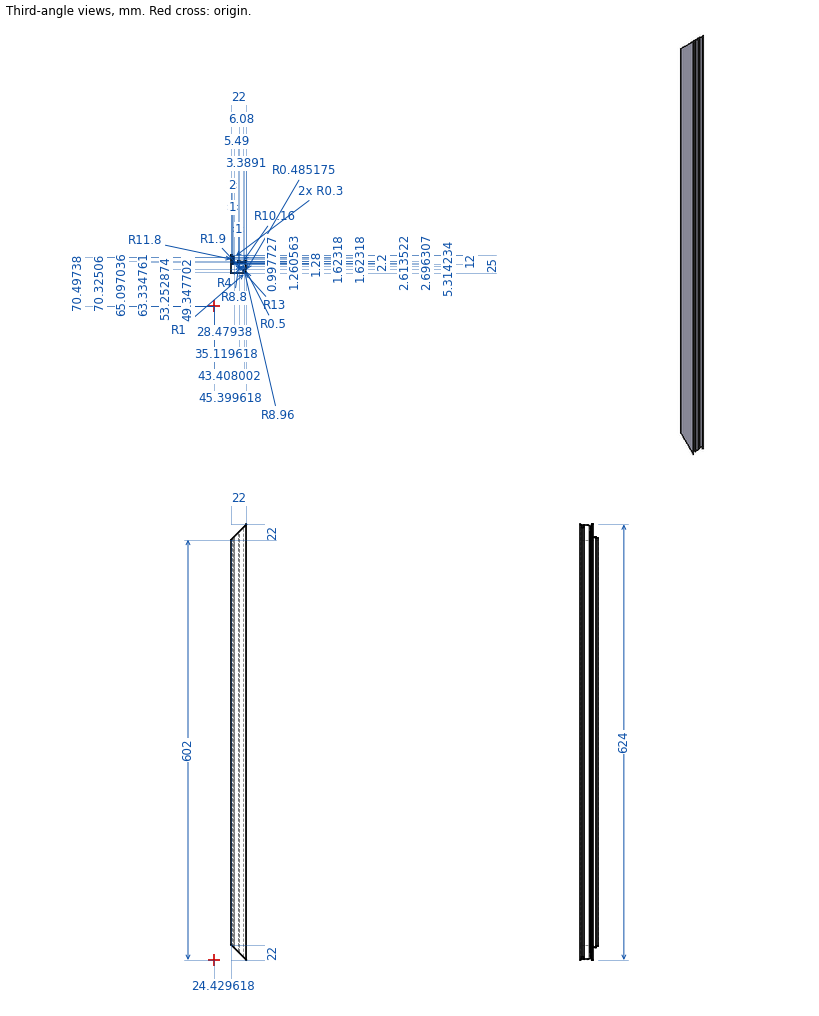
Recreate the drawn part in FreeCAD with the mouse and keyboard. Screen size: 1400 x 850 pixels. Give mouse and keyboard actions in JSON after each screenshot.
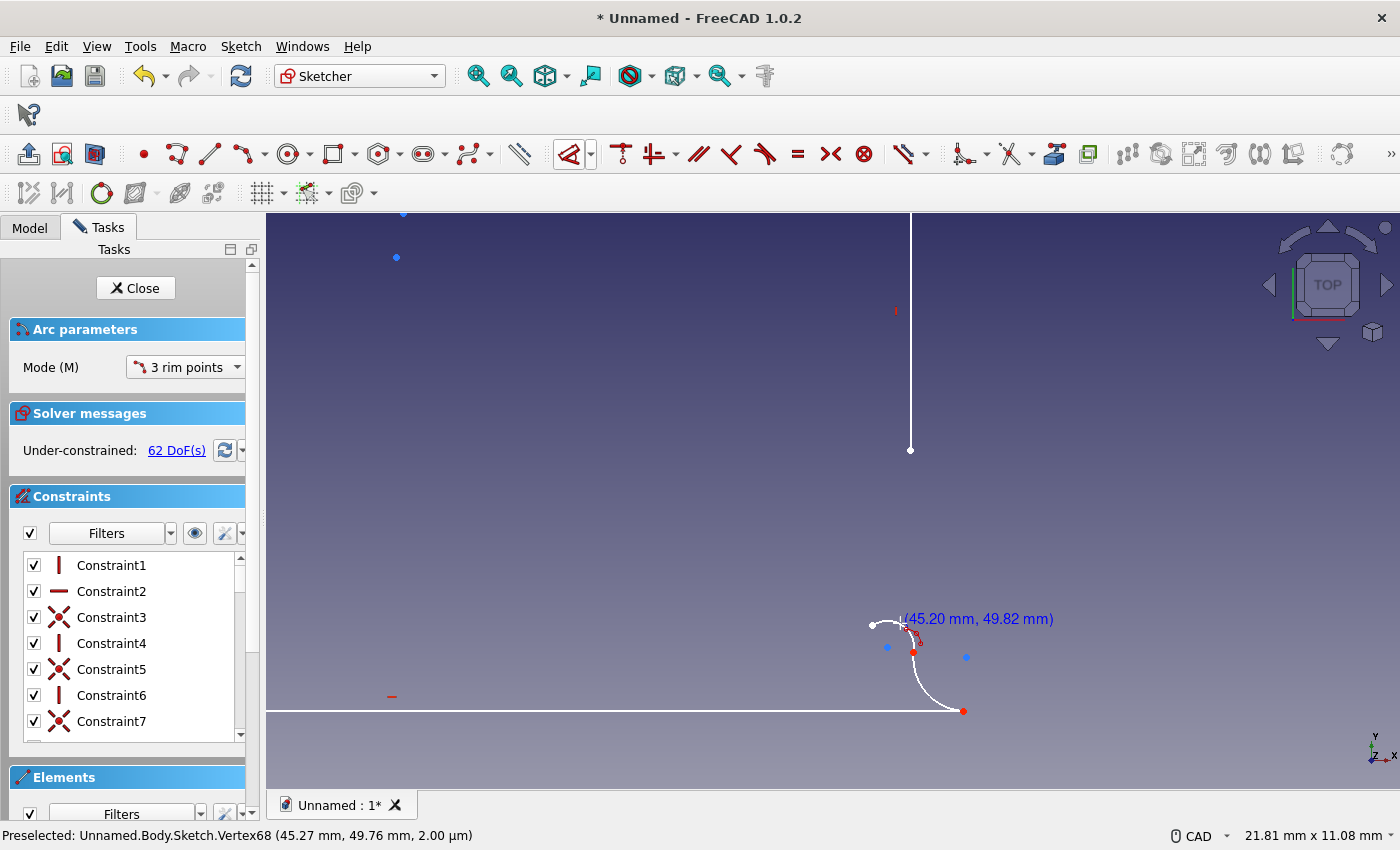
{"action": "left_click", "coordinate": [872, 626]}
{"action": "left_click", "coordinate": [869, 467]}
{"action": "left_click", "coordinate": [713, 549]}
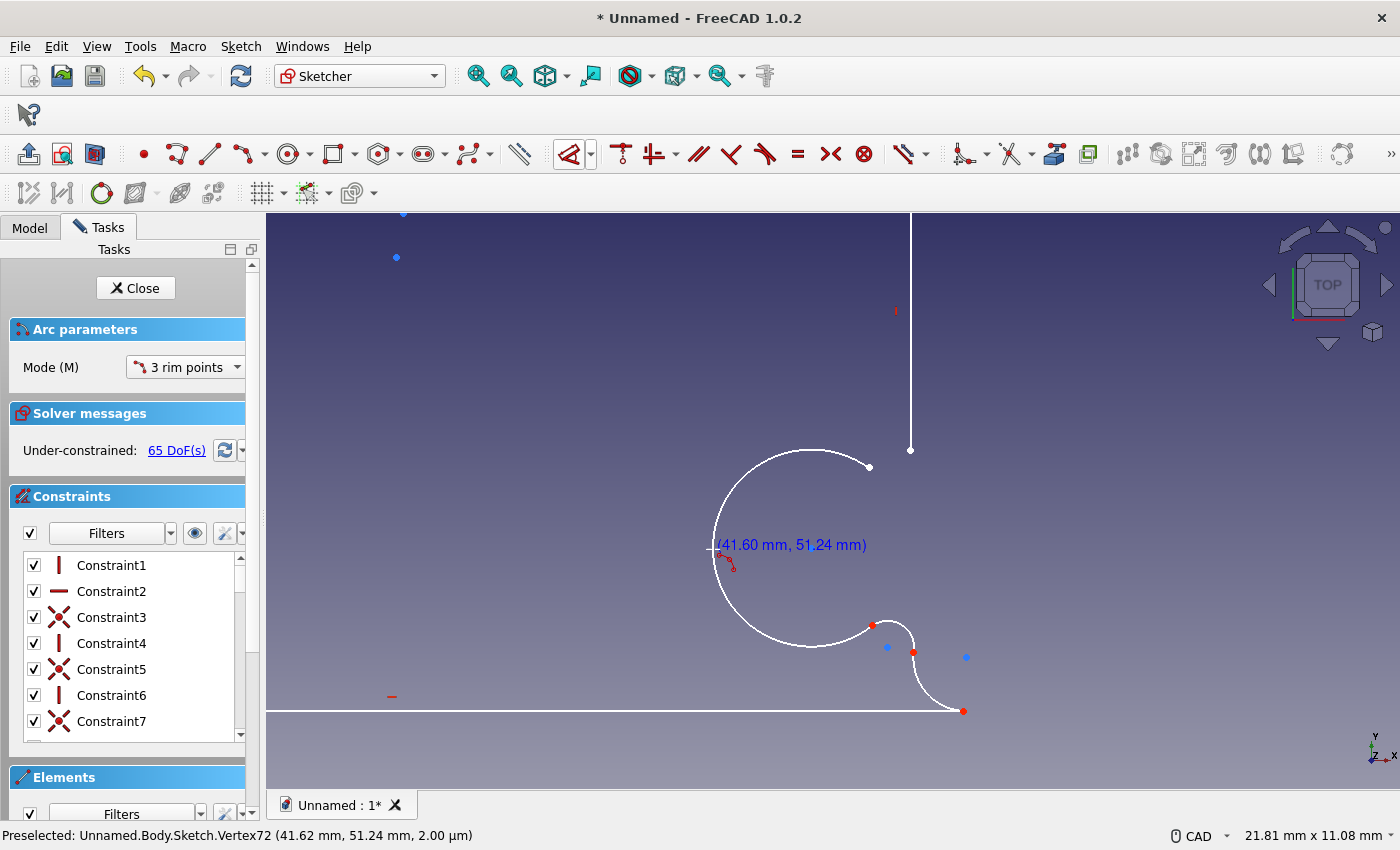
{"action": "left_click", "coordinate": [869, 468]}
{"action": "left_click", "coordinate": [911, 450]}
{"action": "left_click", "coordinate": [896, 469]}
{"action": "key", "text": "Escape"}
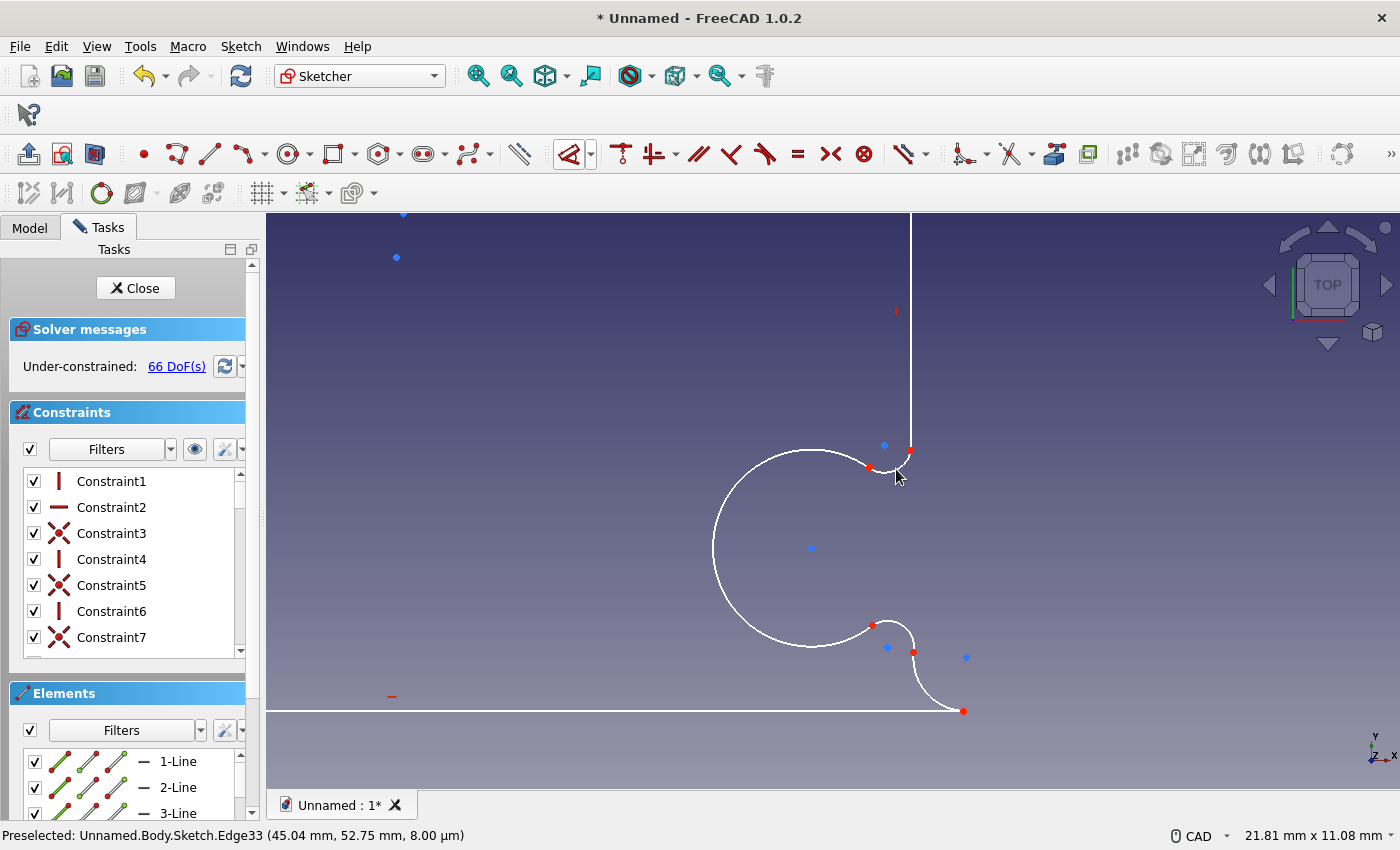
{"action": "left_click", "coordinate": [911, 366]}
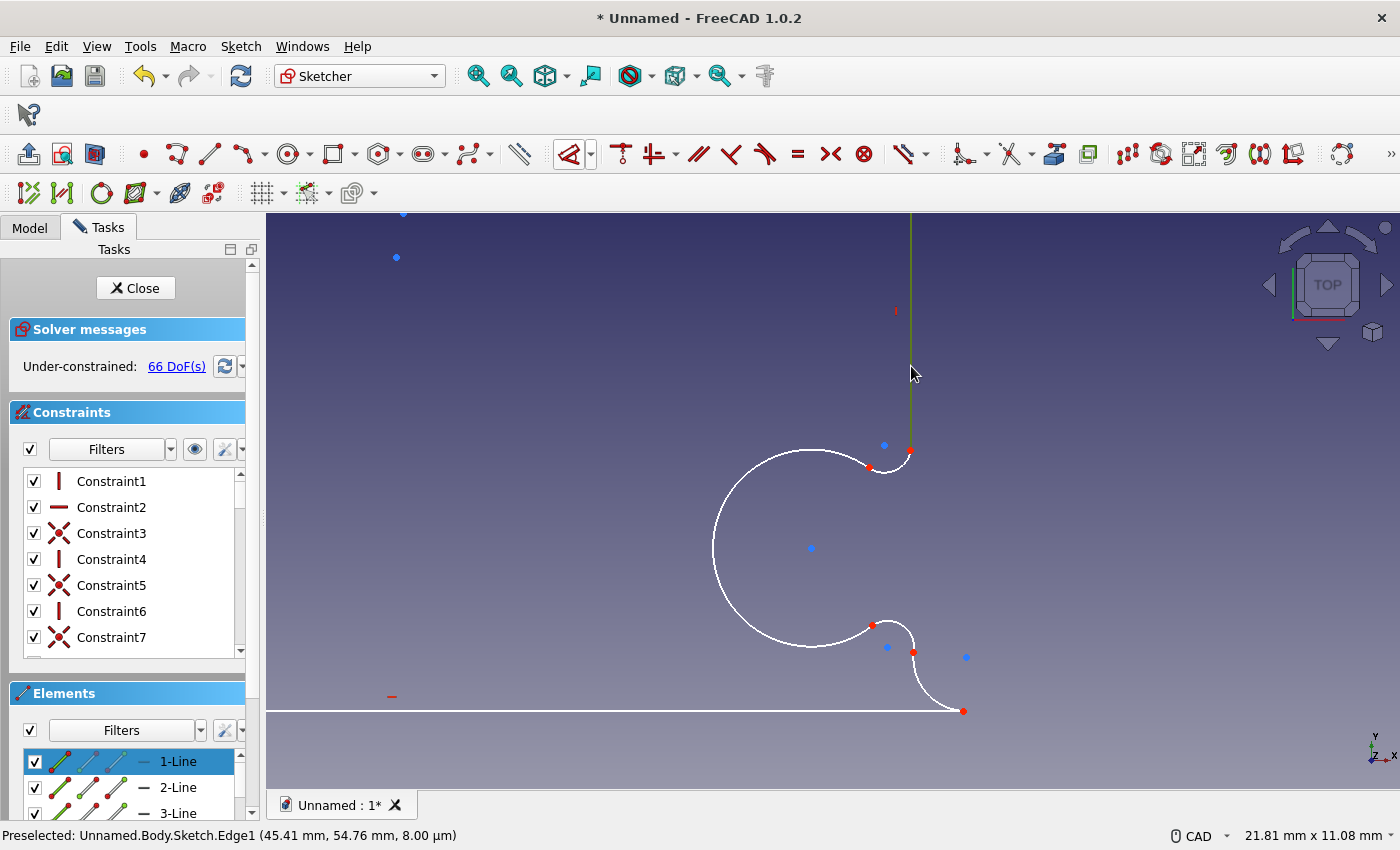
{"action": "scroll", "coordinate": [925, 692], "scroll_direction": "down", "scroll_amount": 6}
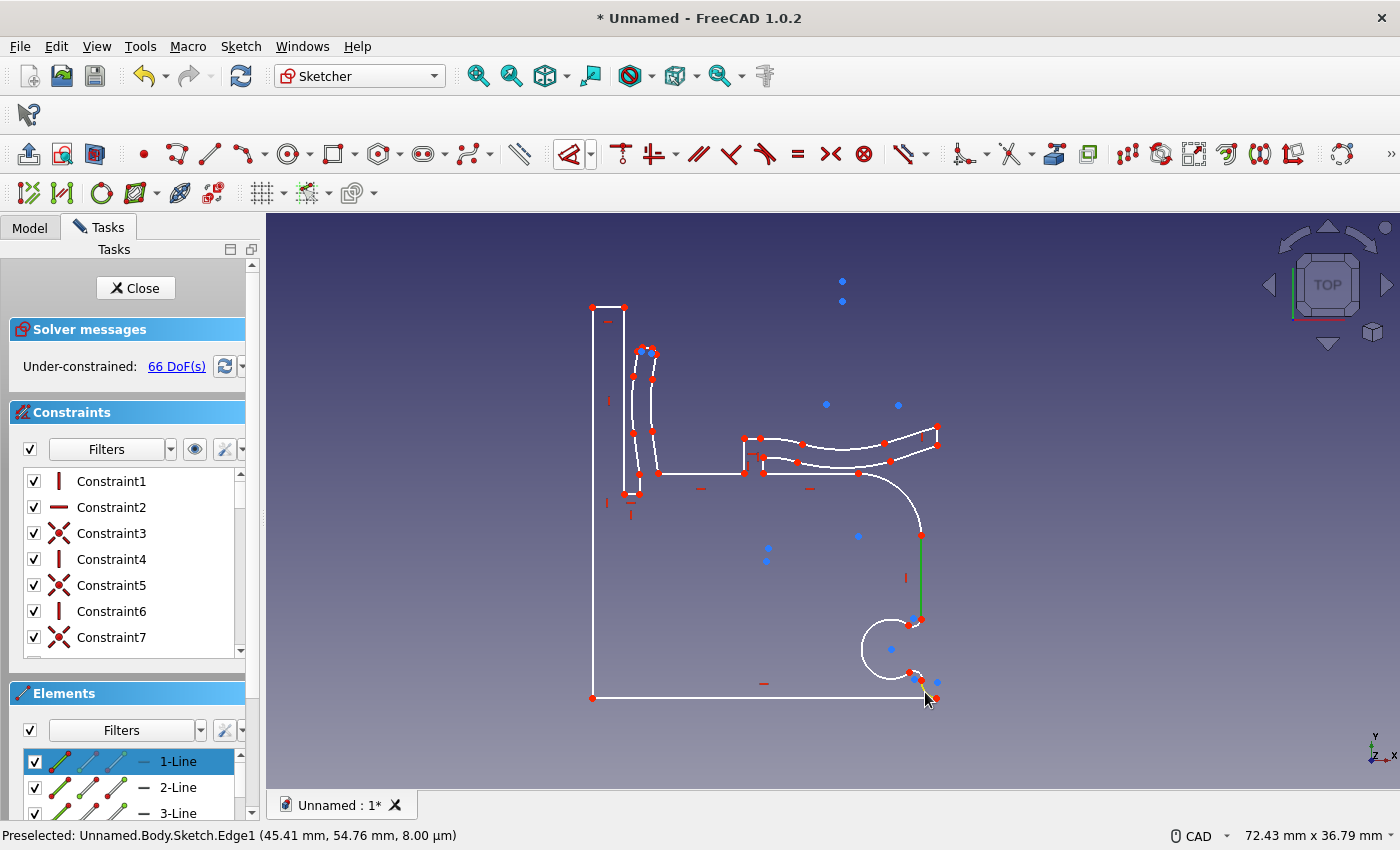
{"action": "left_click", "coordinate": [914, 507]}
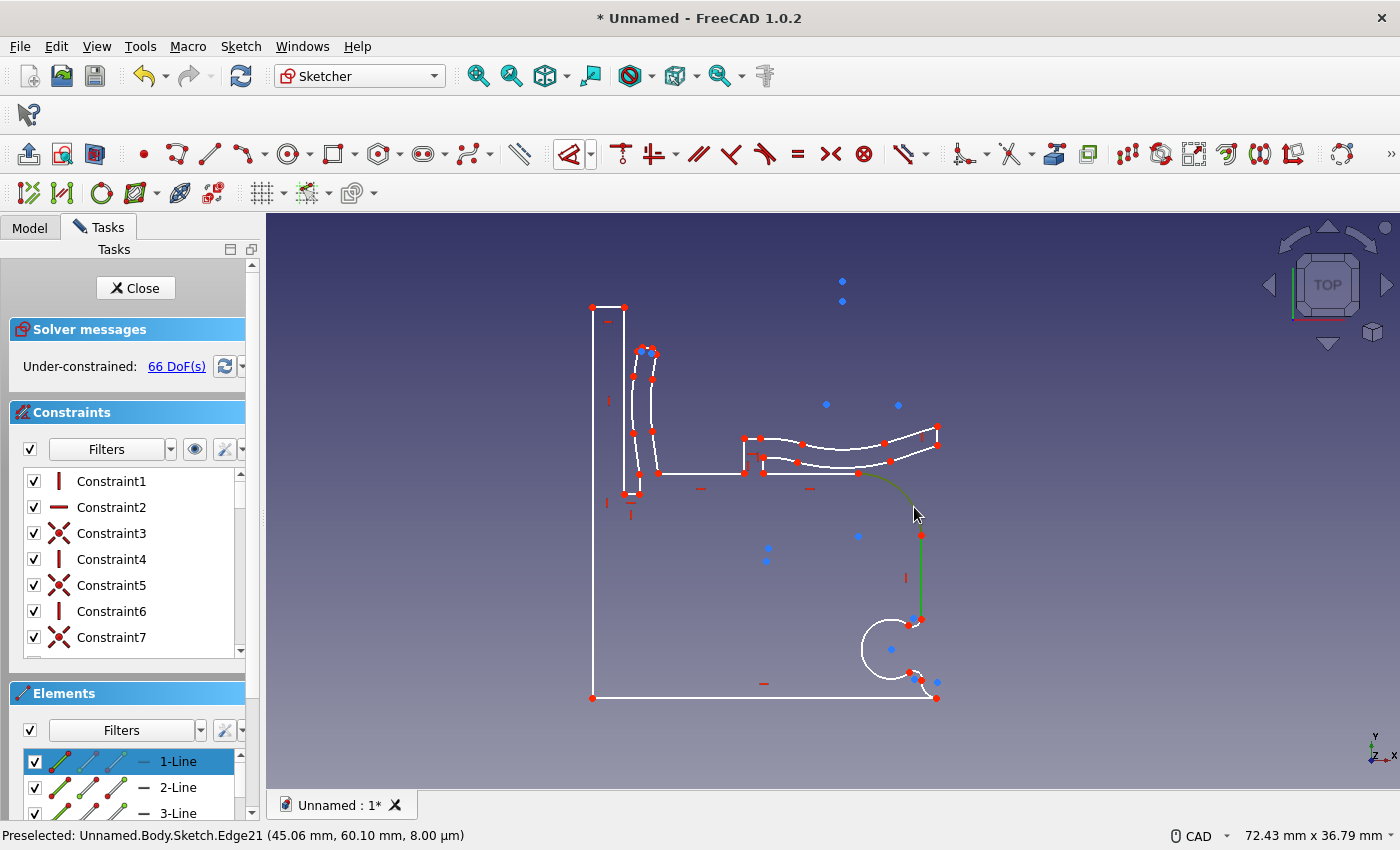
{"action": "key", "text": "t"}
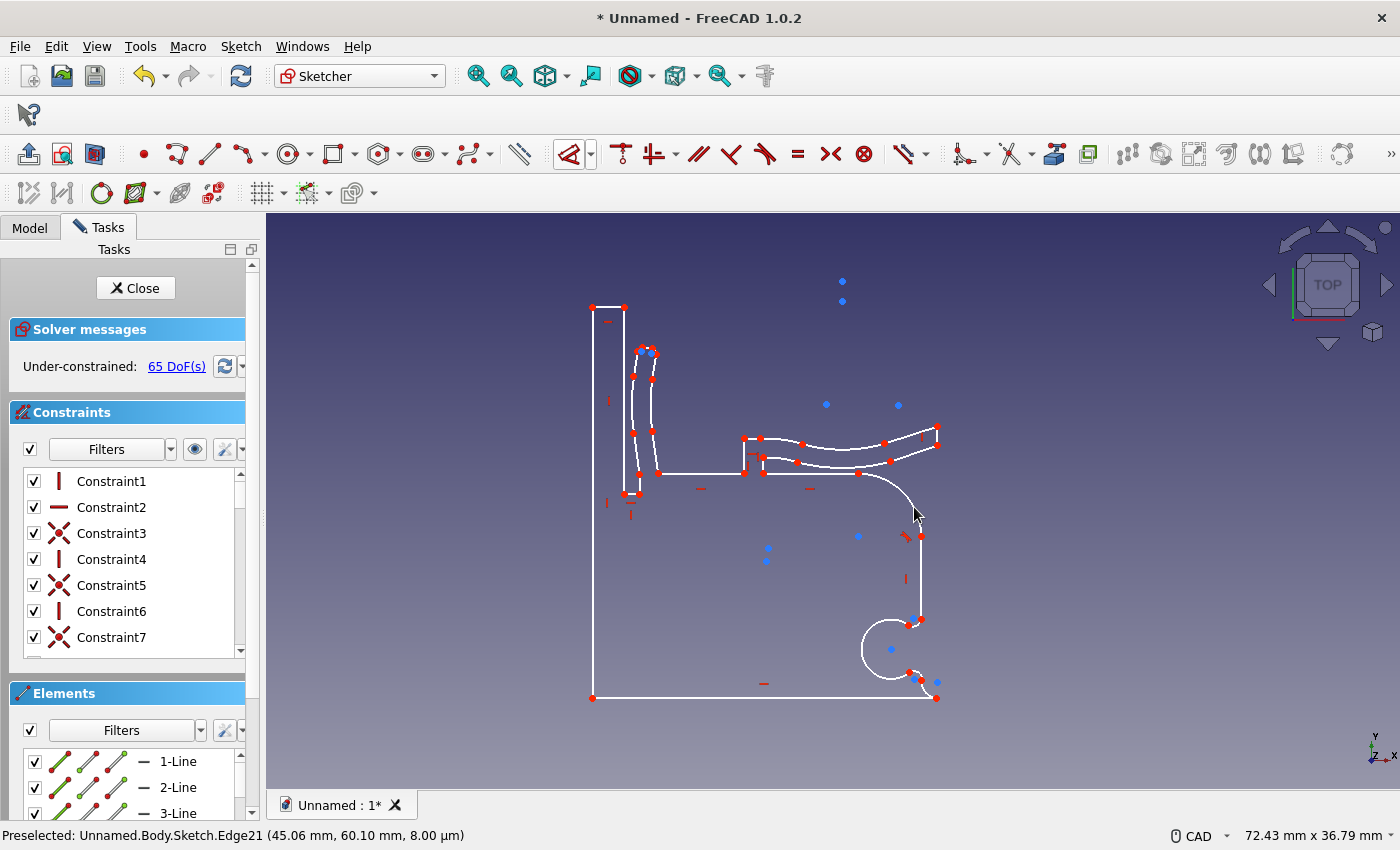
{"action": "left_click", "coordinate": [921, 595]}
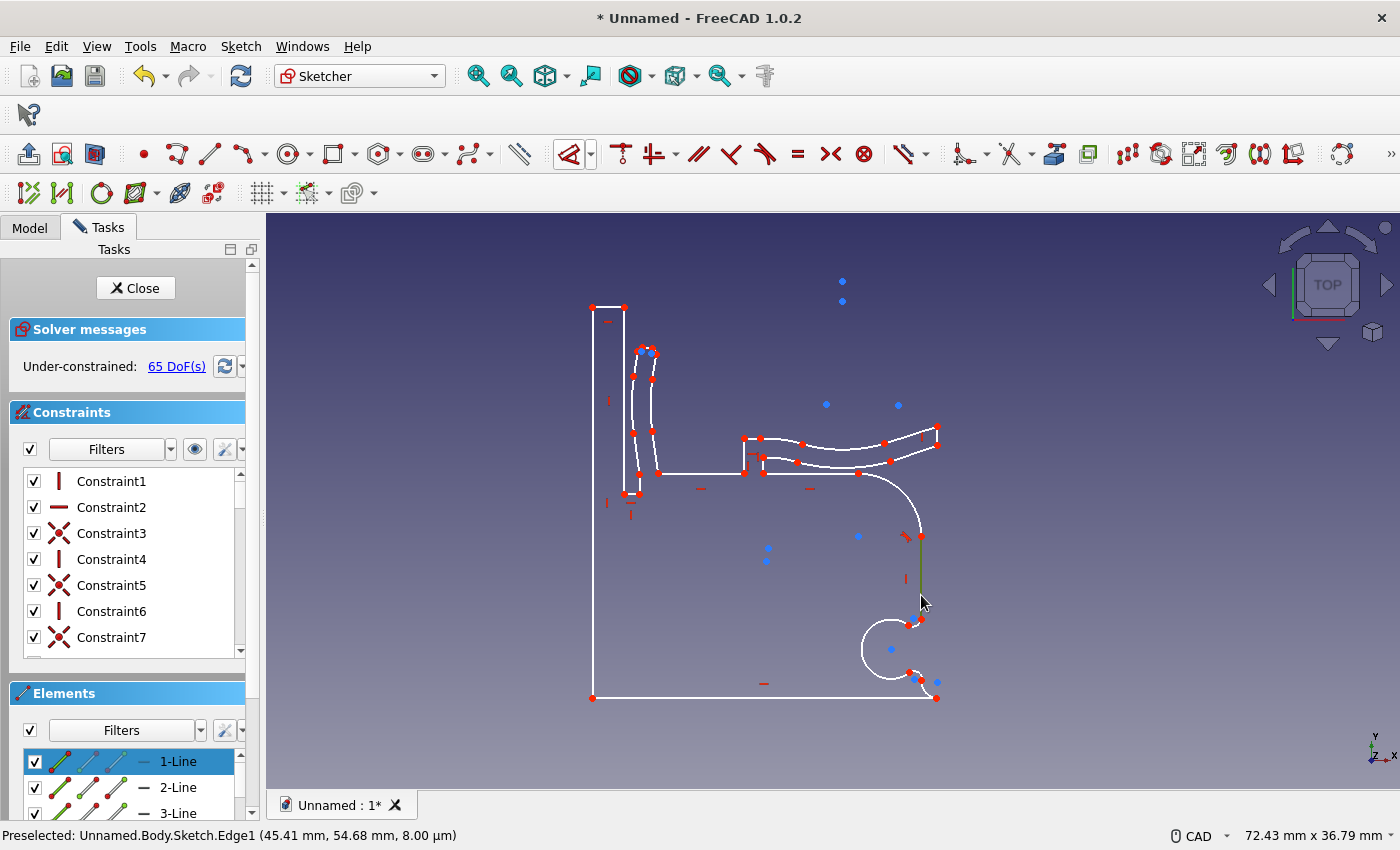
{"action": "scroll", "coordinate": [916, 626], "scroll_direction": "up", "scroll_amount": 3}